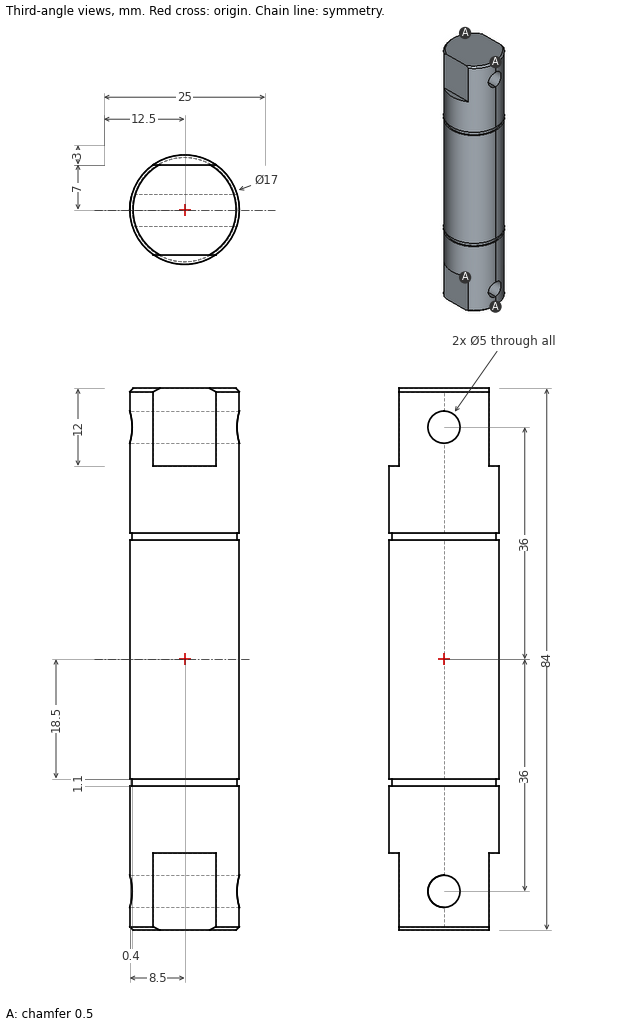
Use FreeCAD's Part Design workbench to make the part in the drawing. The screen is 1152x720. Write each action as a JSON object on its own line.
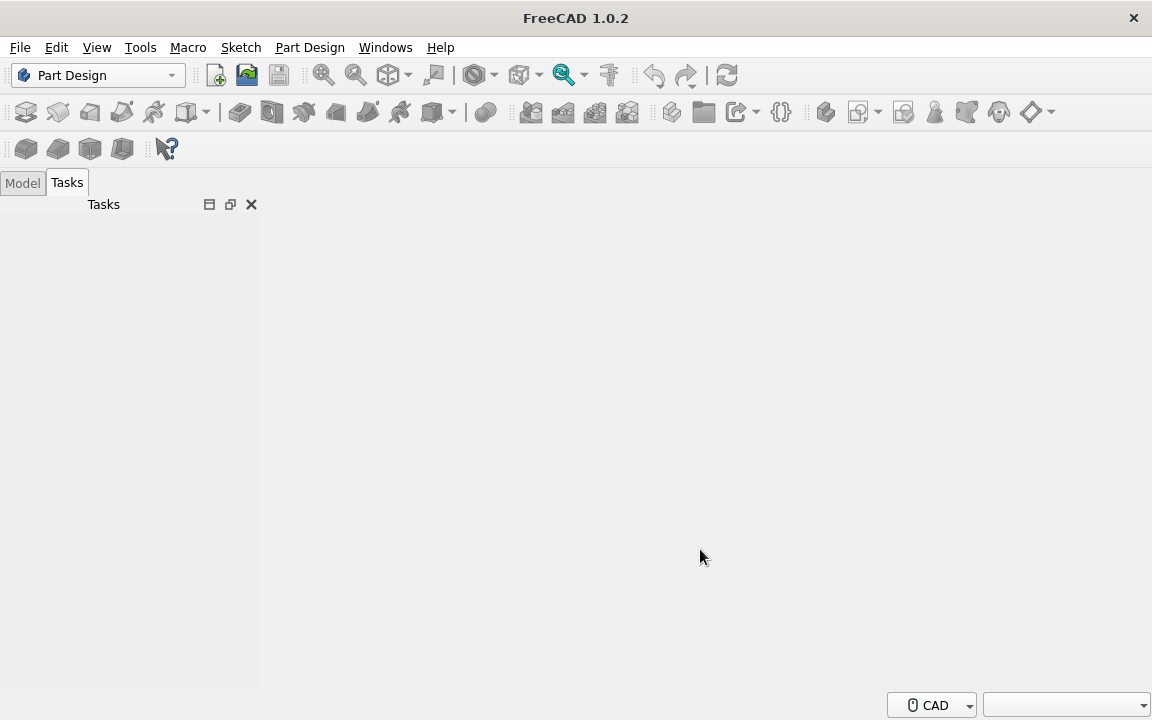
{"action": "left_click", "coordinate": [216, 76]}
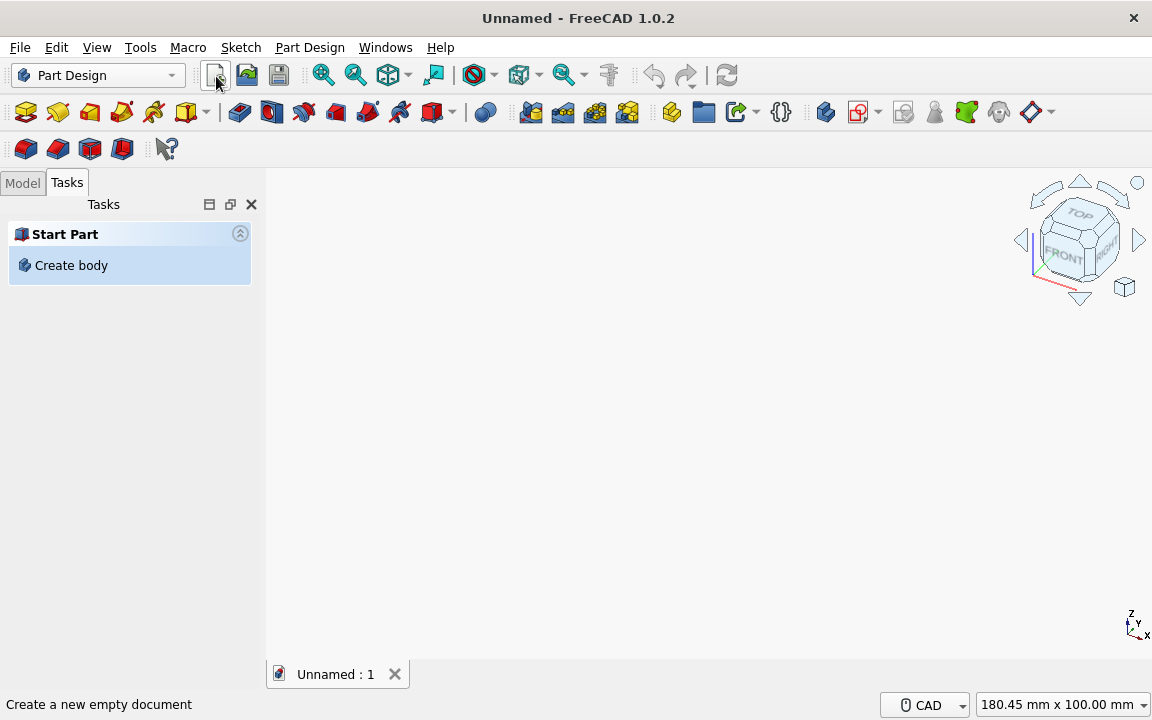
{"action": "left_click", "coordinate": [858, 112]}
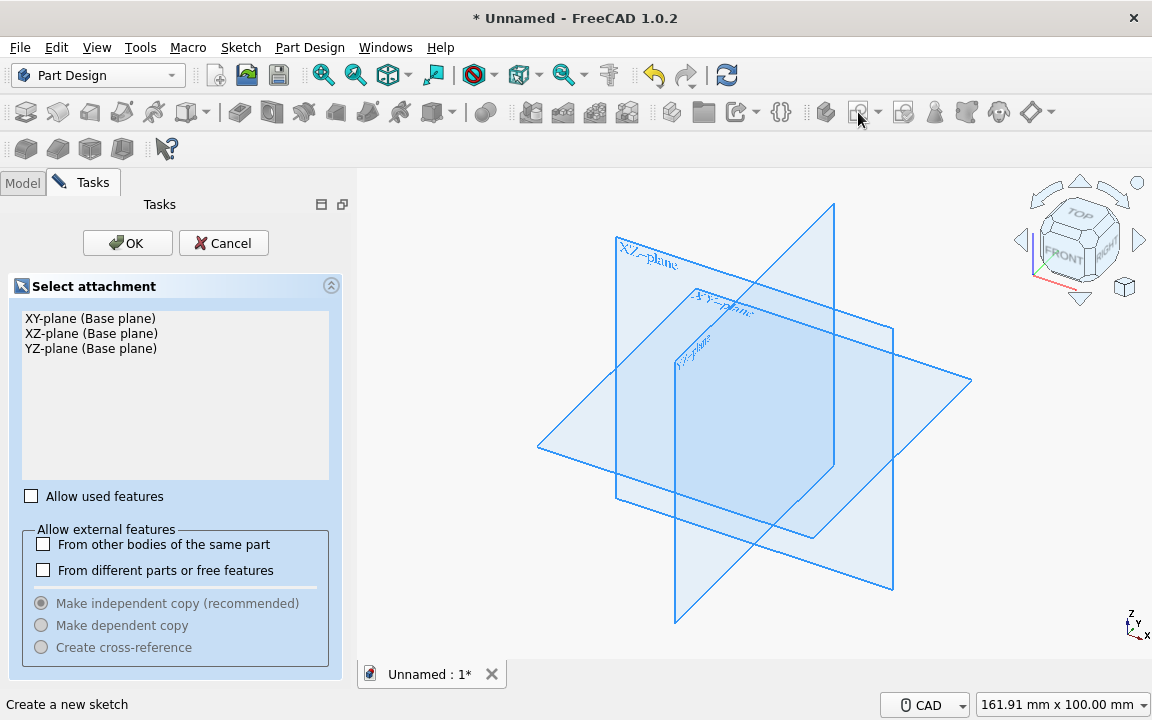
{"action": "left_click", "coordinate": [82, 318]}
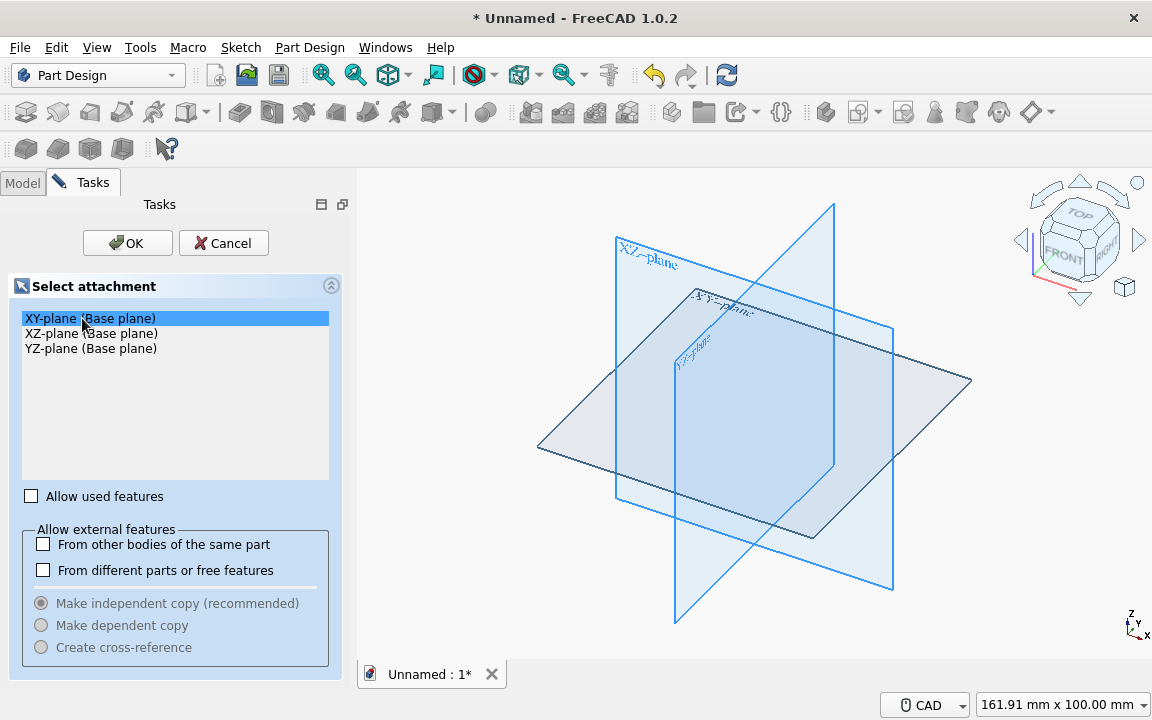
{"action": "left_click", "coordinate": [128, 243]}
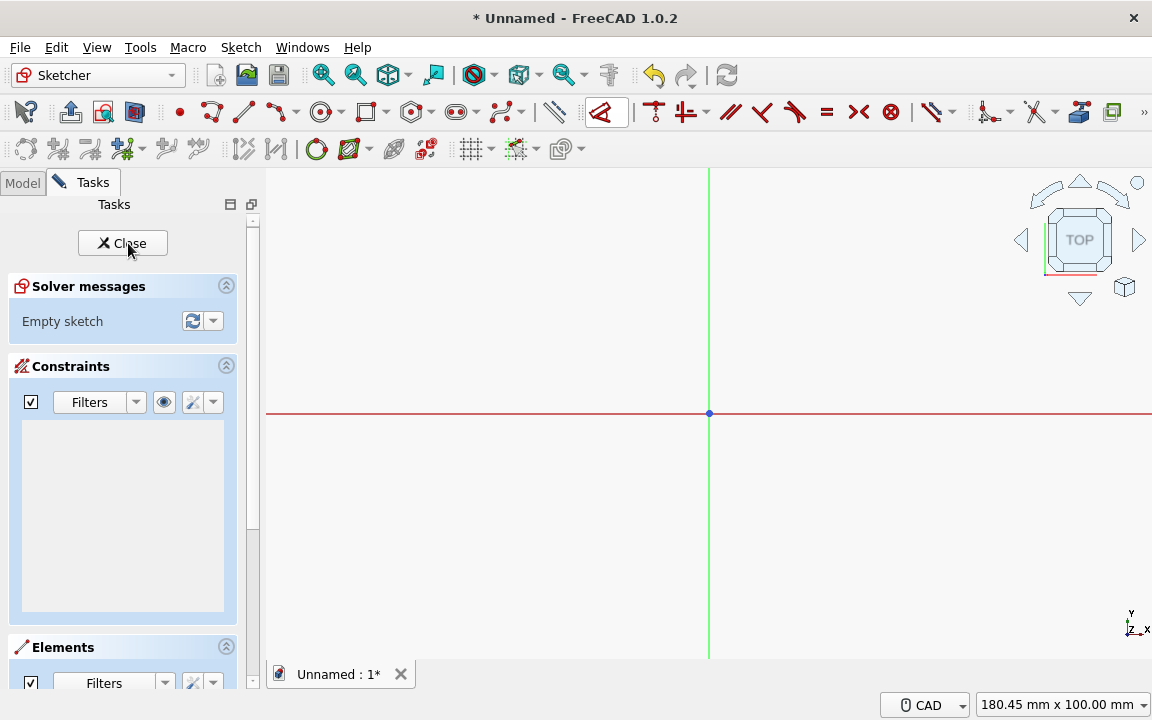
{"action": "scroll", "coordinate": [731, 414], "scroll_direction": "up", "scroll_amount": 7}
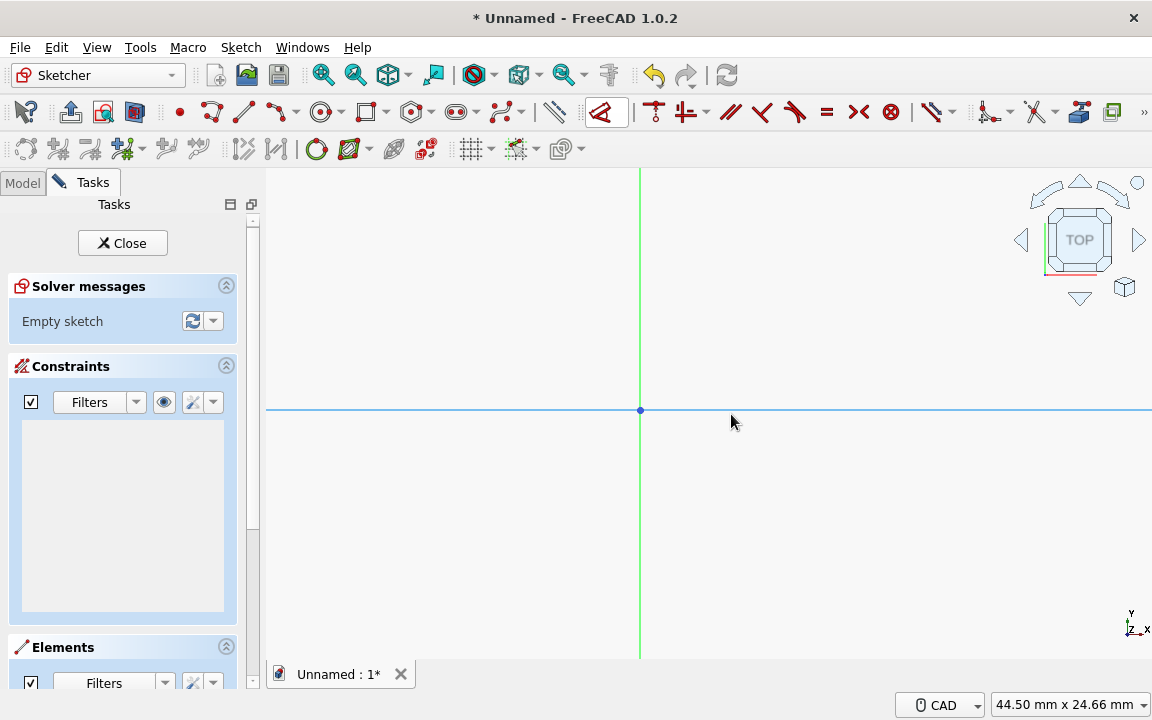
{"action": "left_click", "coordinate": [322, 112]}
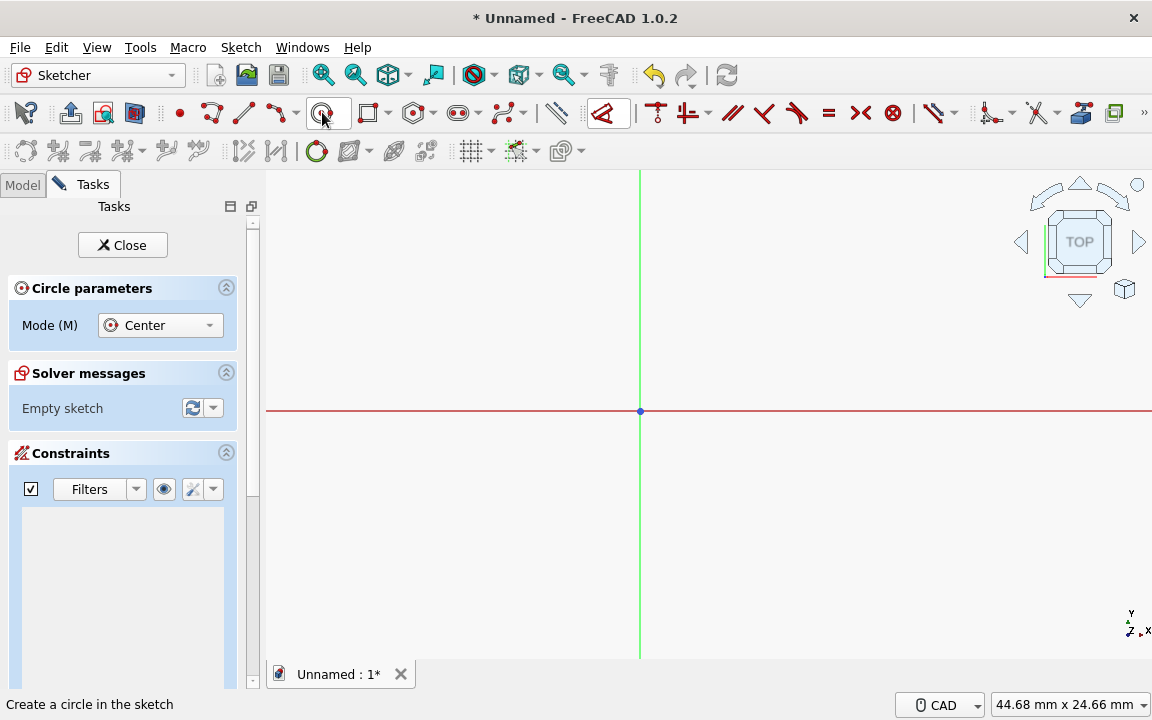
{"action": "left_click", "coordinate": [640, 411]}
{"action": "left_click", "coordinate": [760, 292]}
{"action": "key", "text": "Escape"}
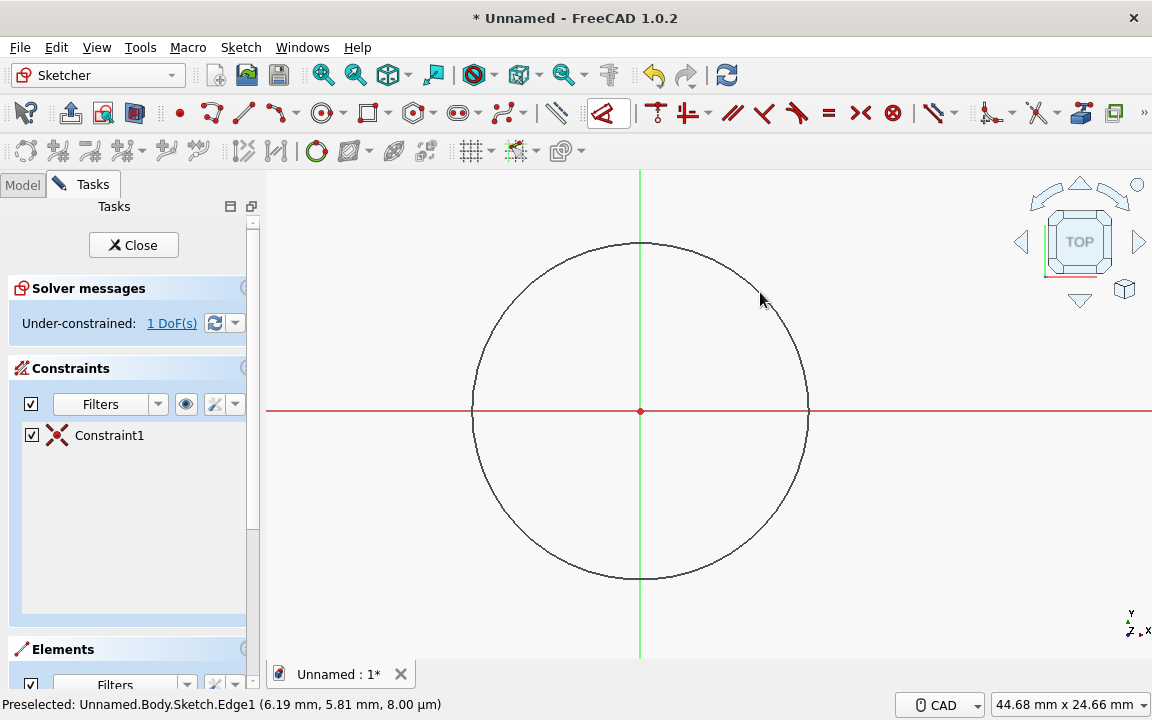
{"action": "left_click", "coordinate": [602, 114]}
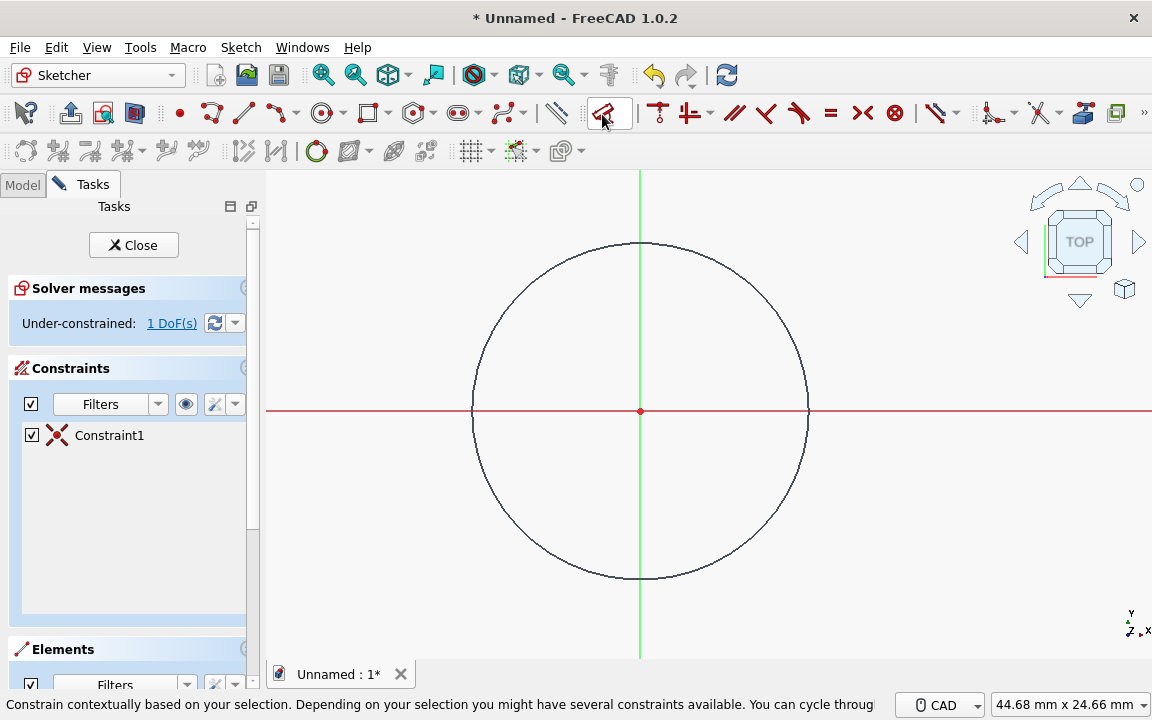
{"action": "left_click", "coordinate": [759, 292]}
{"action": "left_click", "coordinate": [782, 269]}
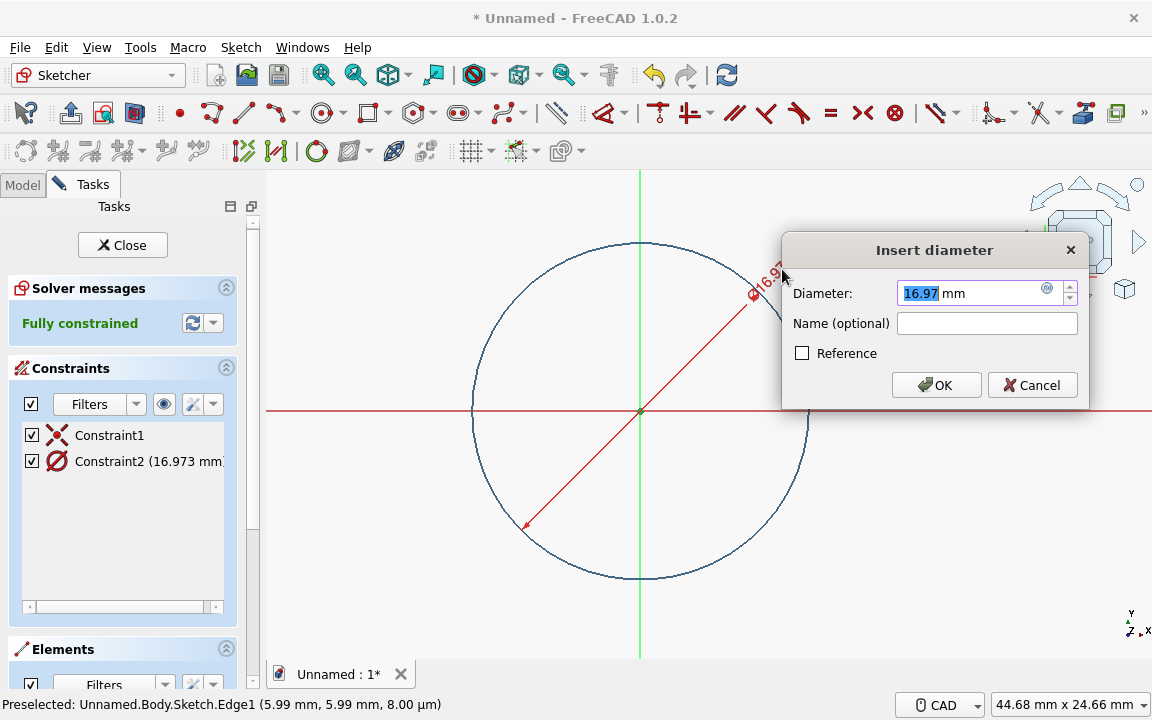
{"action": "type", "text": "17"}
{"action": "key", "text": "Return"}
{"action": "key", "text": "Escape"}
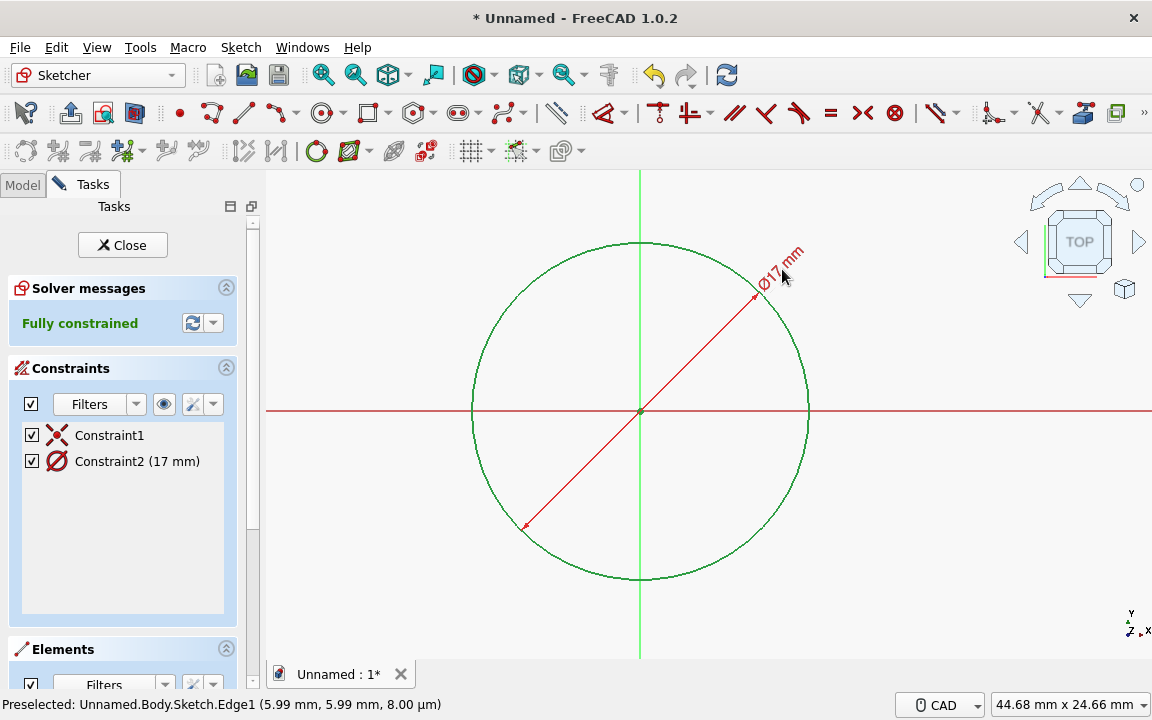
{"action": "left_click", "coordinate": [123, 245]}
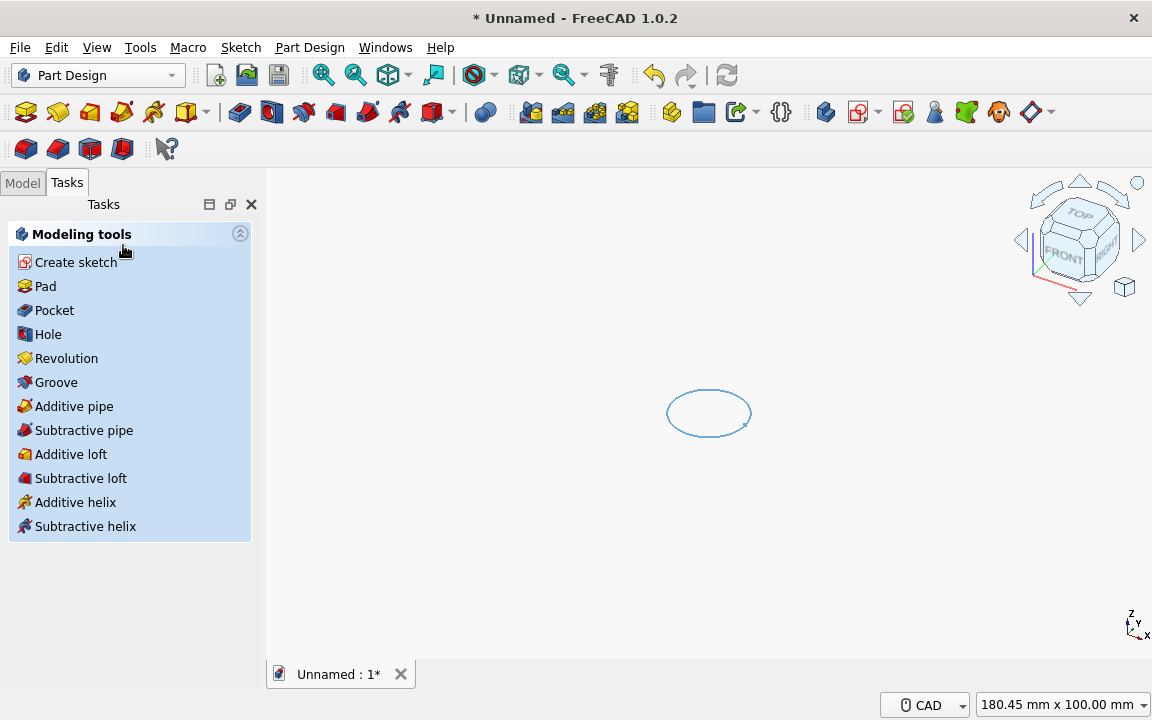
{"action": "left_click", "coordinate": [26, 112]}